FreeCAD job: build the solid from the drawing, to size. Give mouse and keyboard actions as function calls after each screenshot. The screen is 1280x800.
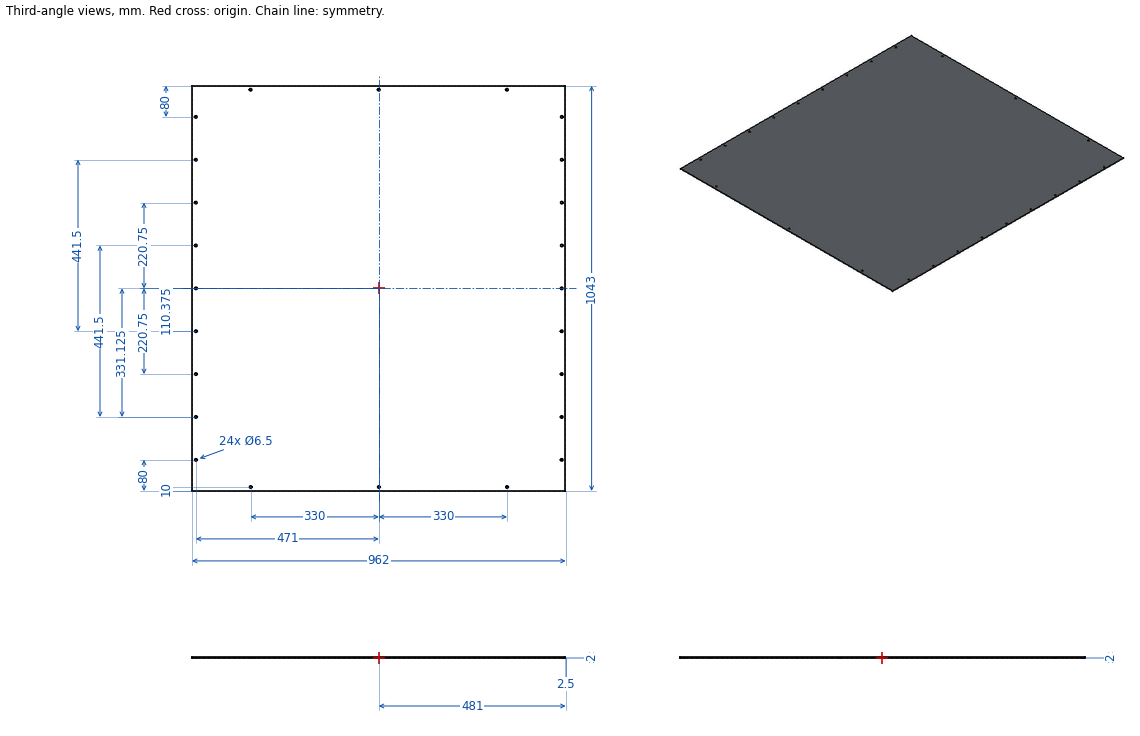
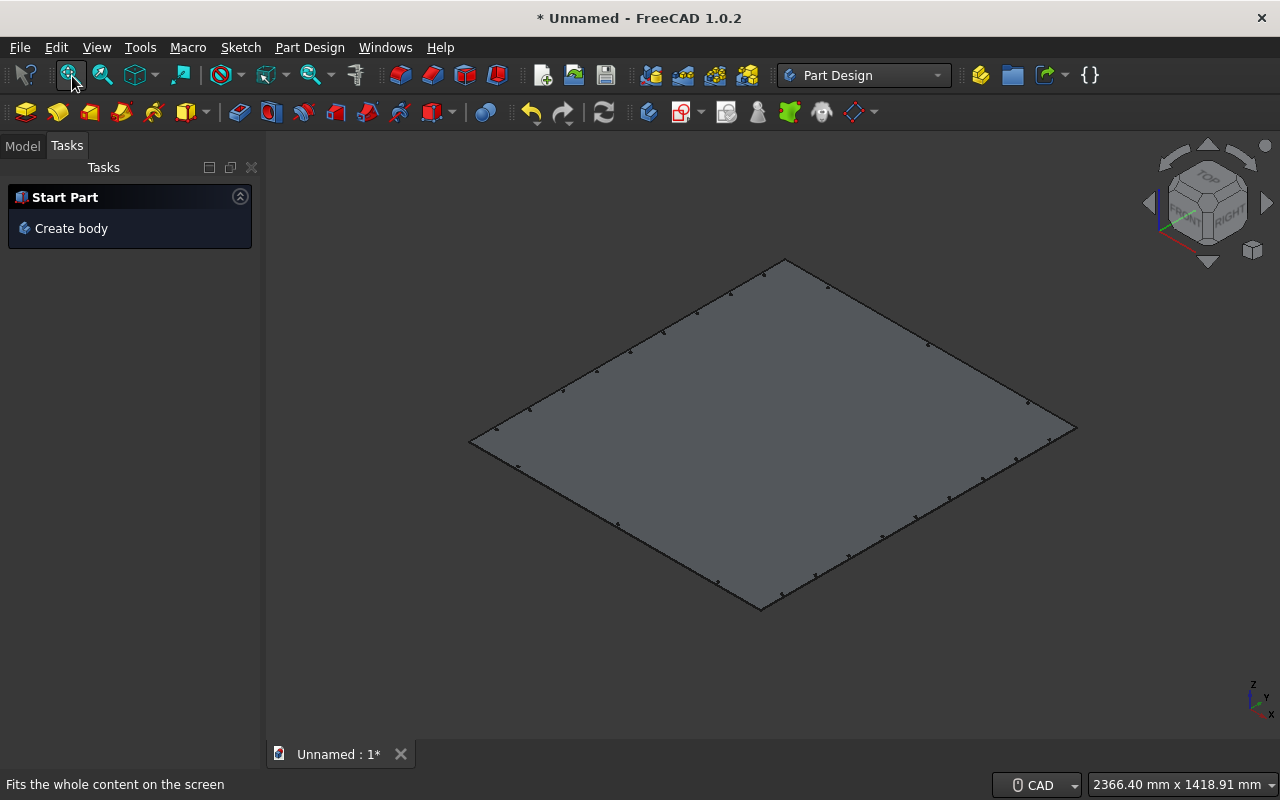
scroll(740, 597, up, 15)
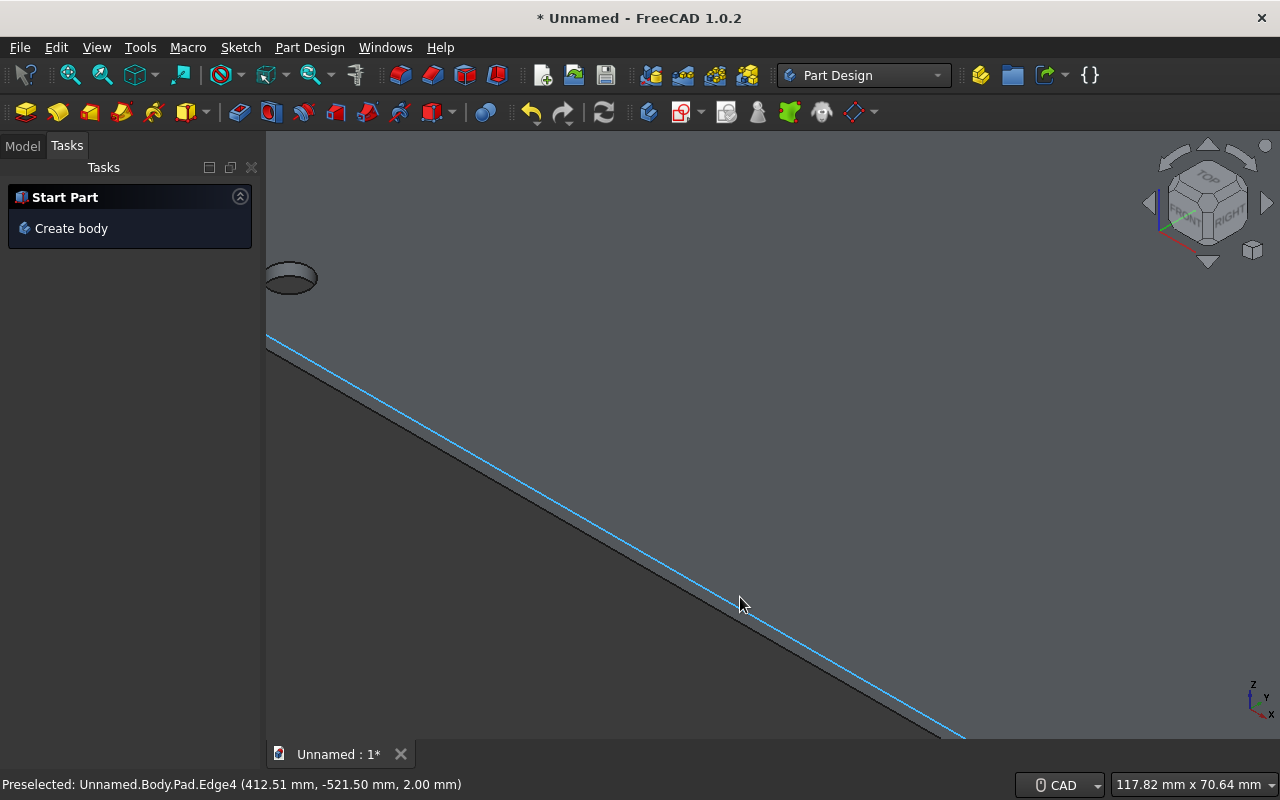
key(v)
key(f)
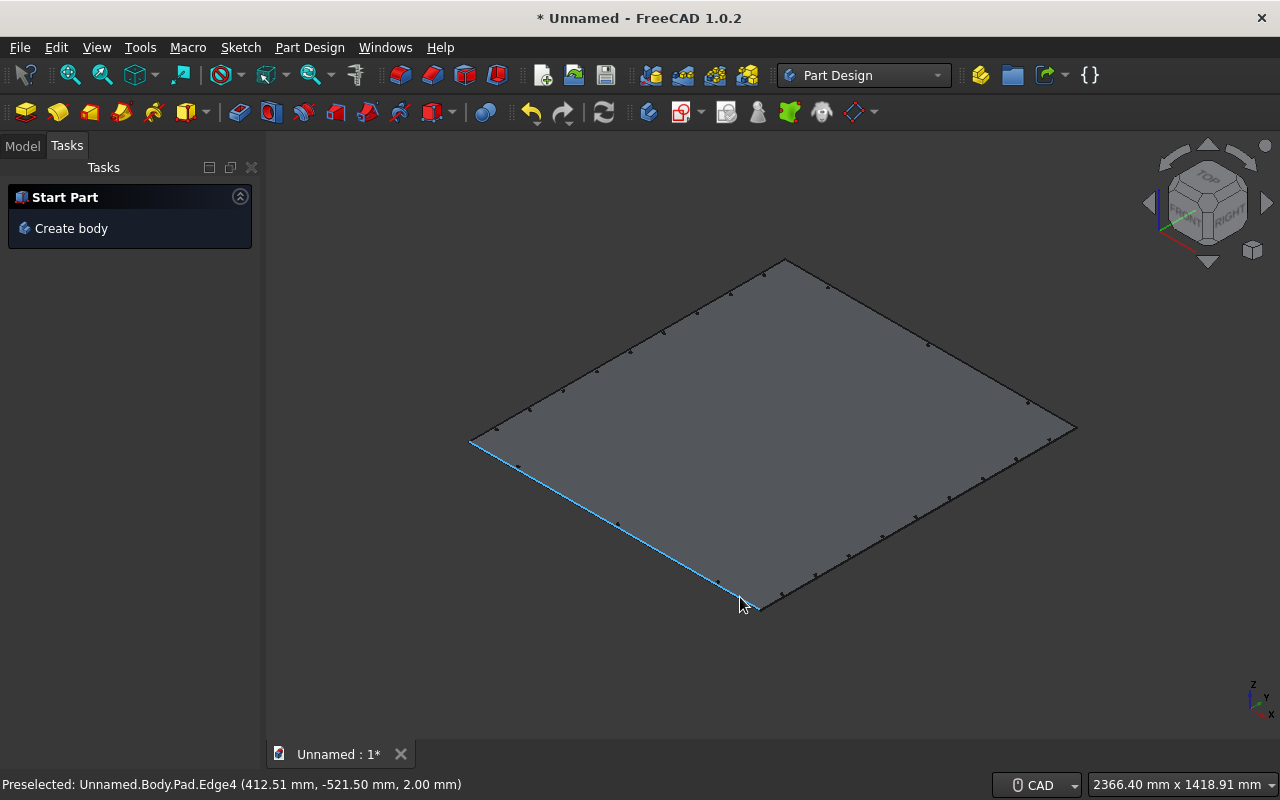
key(1)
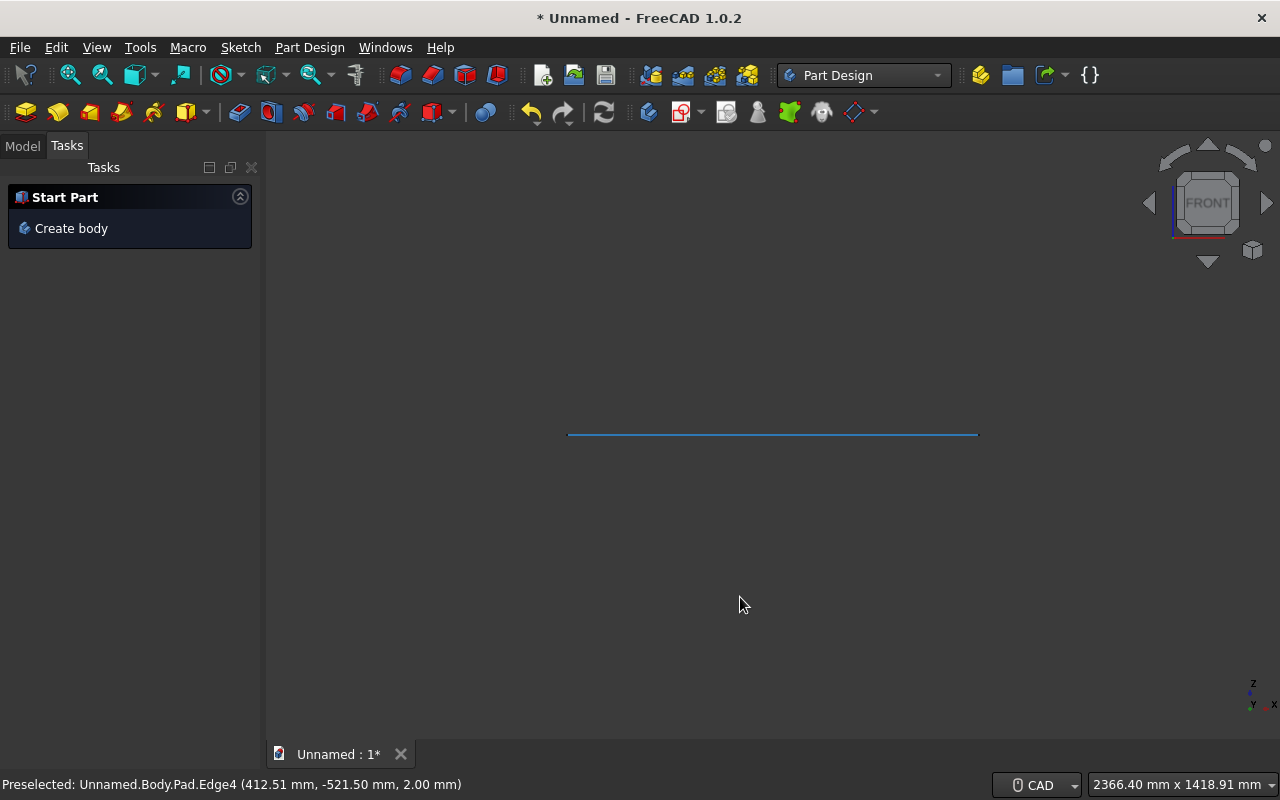
click(72, 76)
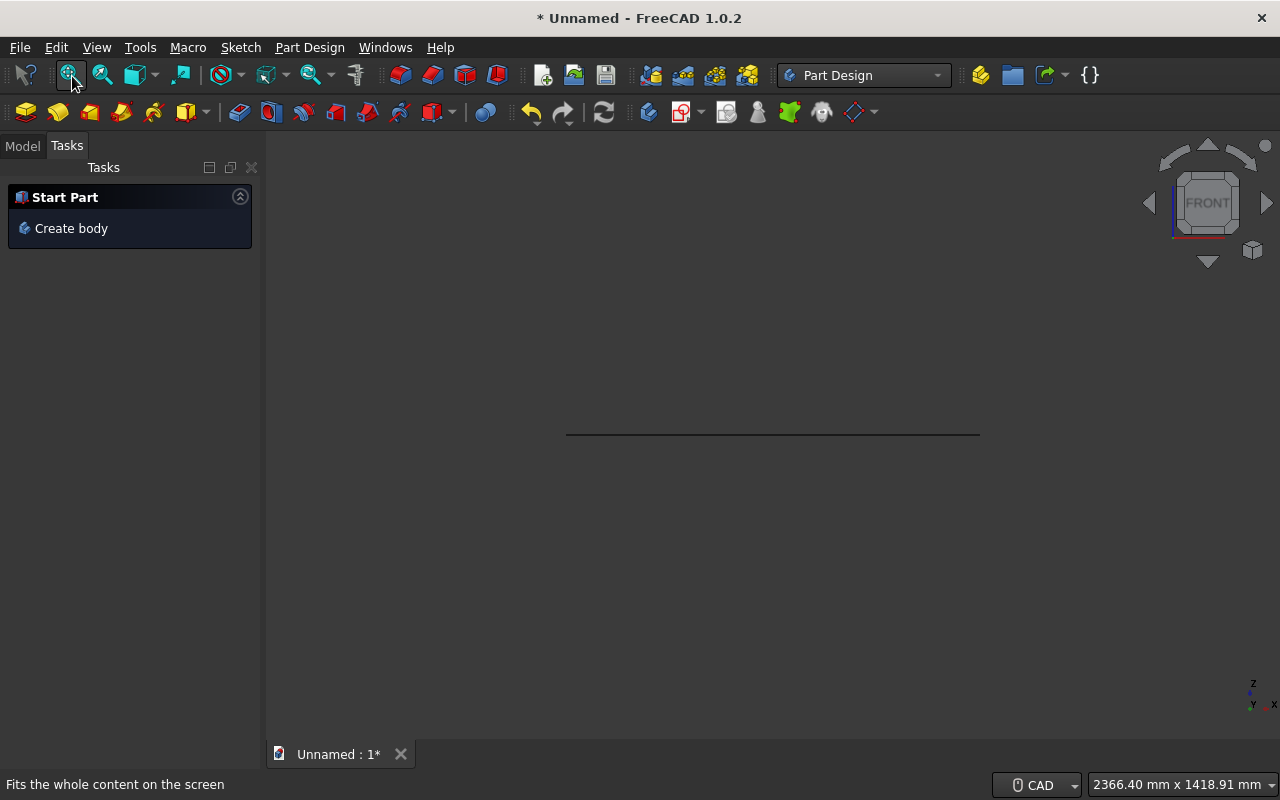
scroll(950, 434, up, 15)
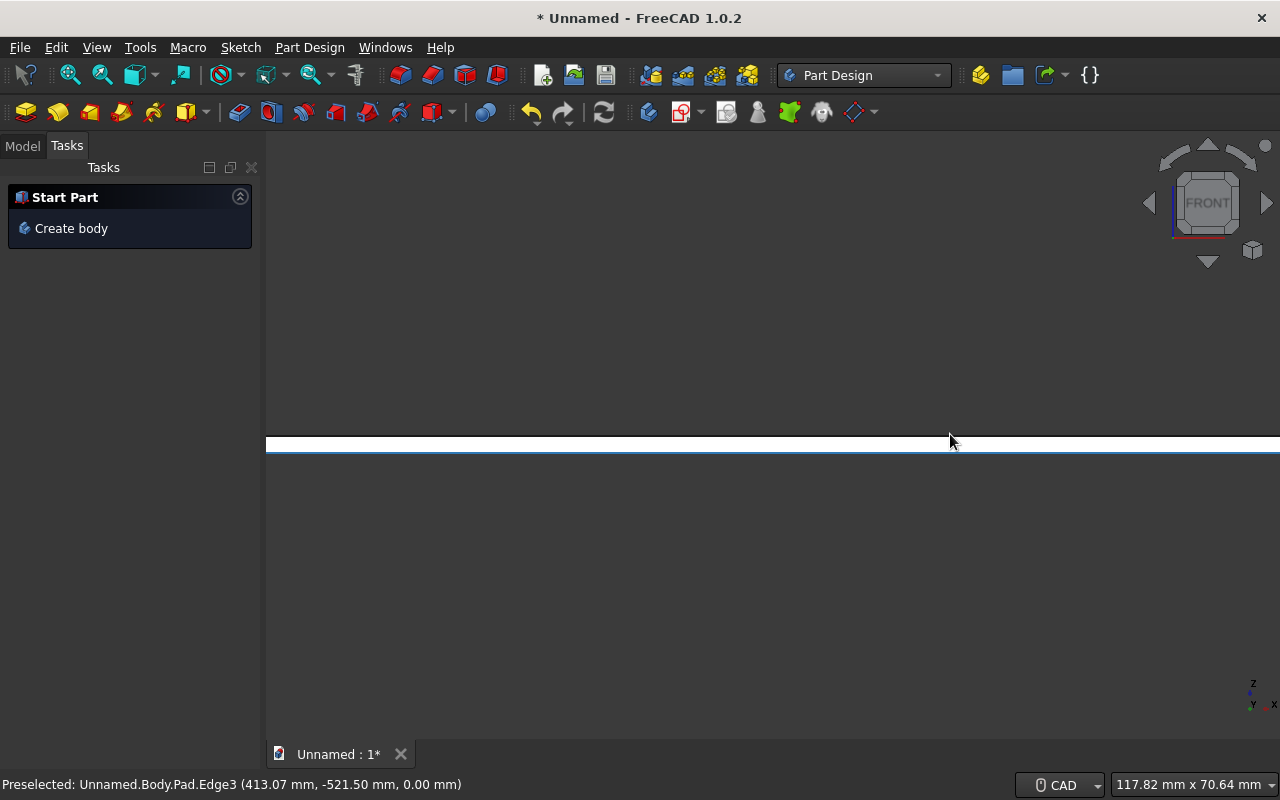
click(930, 444)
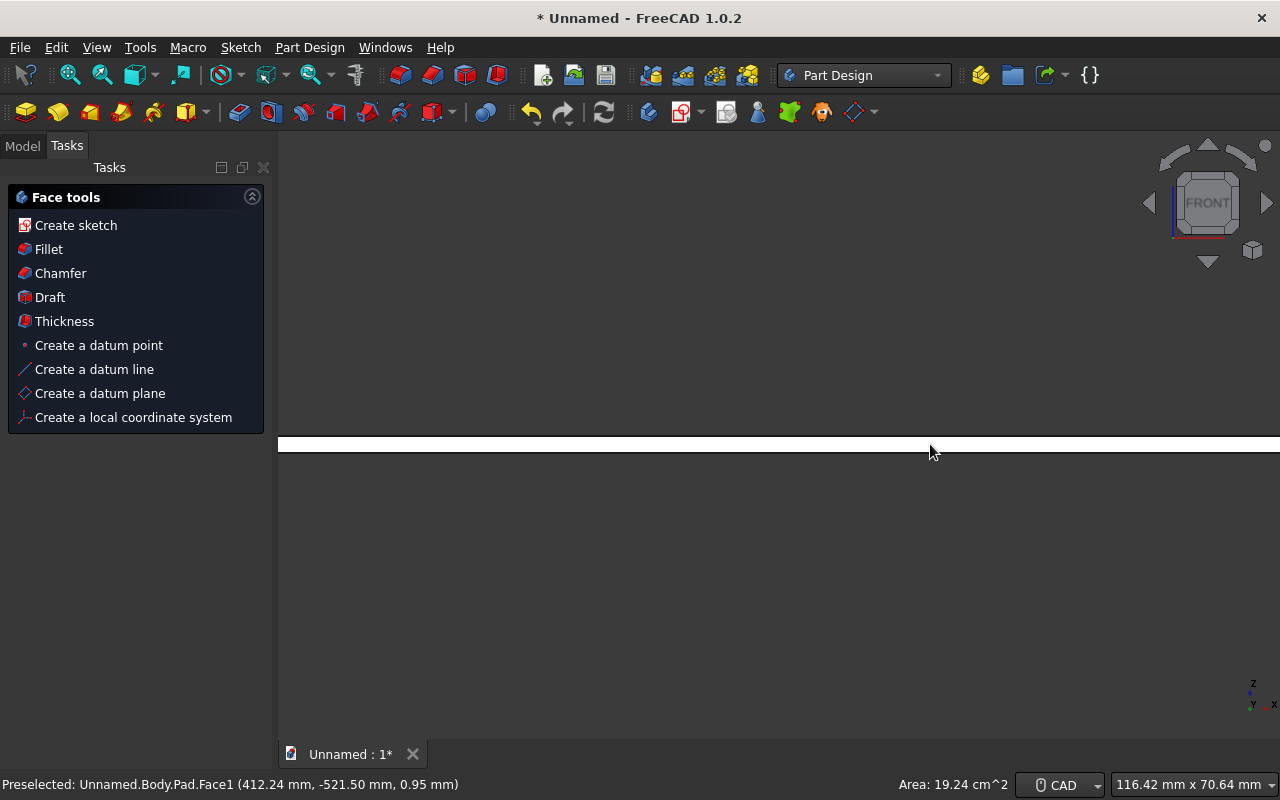
click(682, 112)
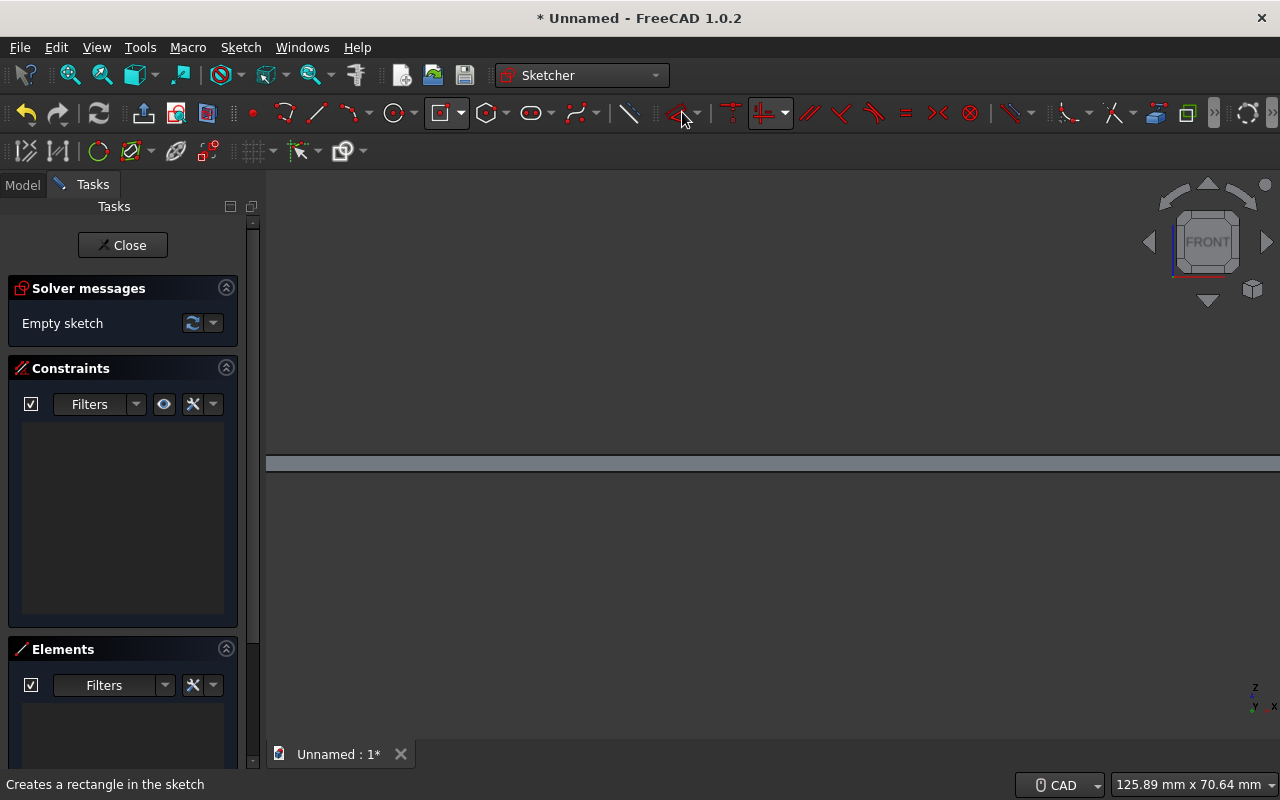
scroll(704, 454, down, 5)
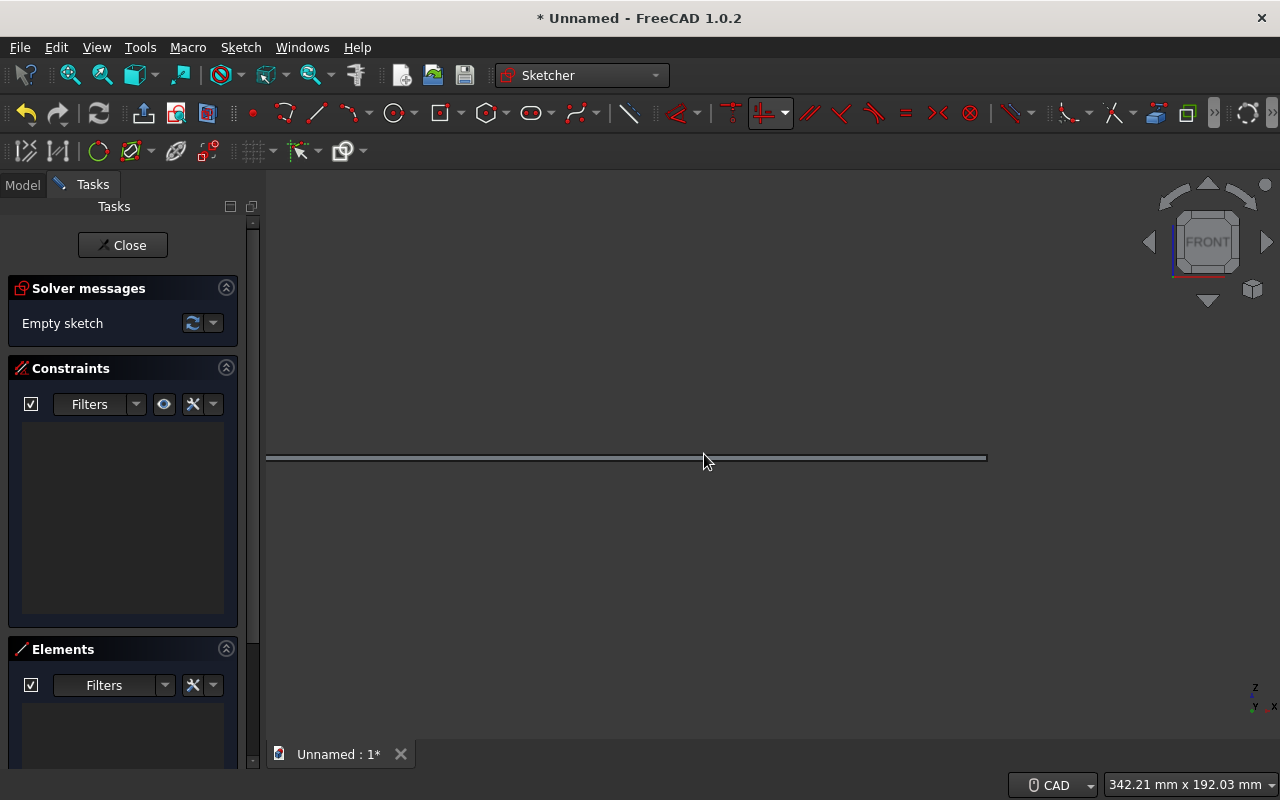
scroll(998, 458, up, 15)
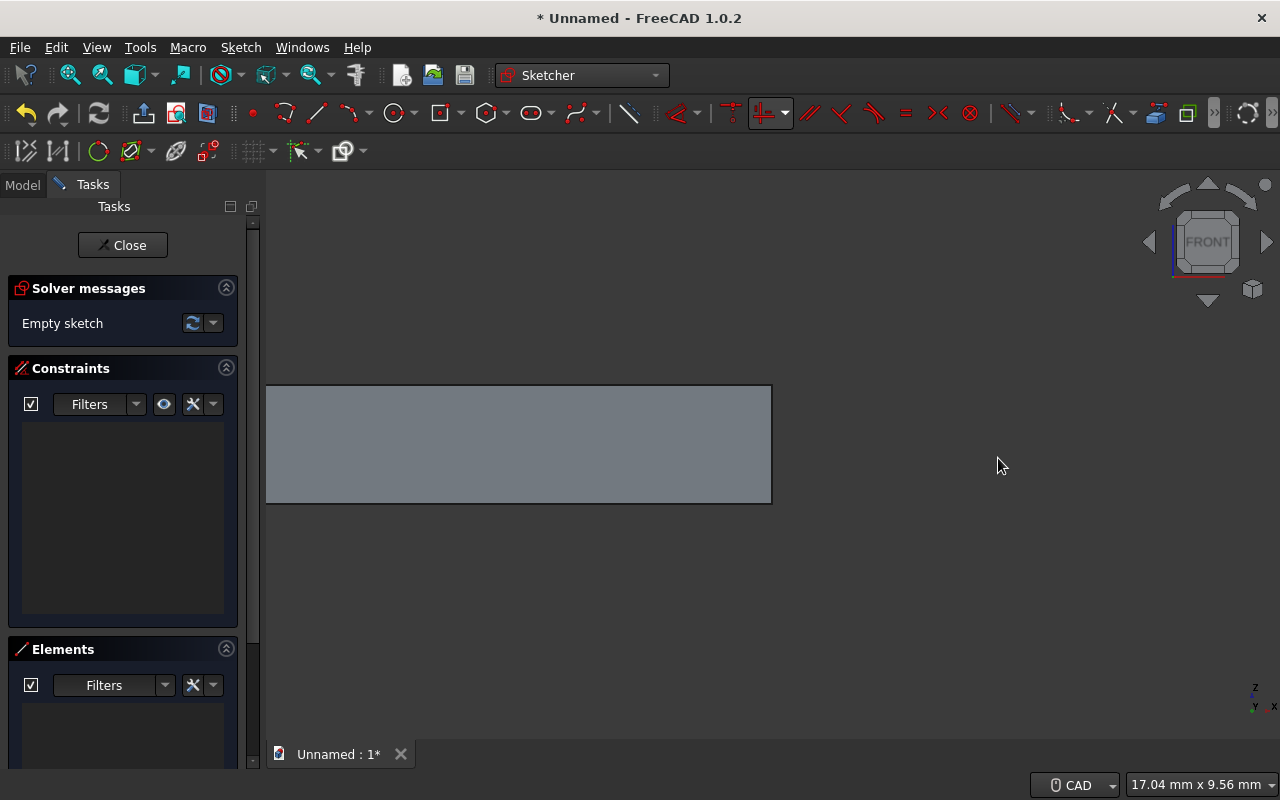
scroll(695, 440, up, 6)